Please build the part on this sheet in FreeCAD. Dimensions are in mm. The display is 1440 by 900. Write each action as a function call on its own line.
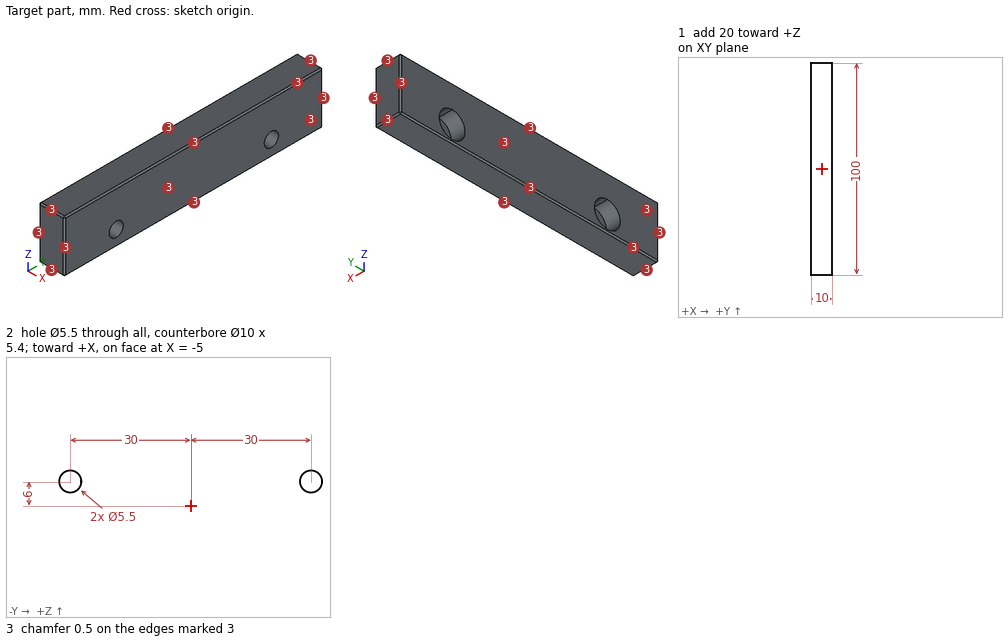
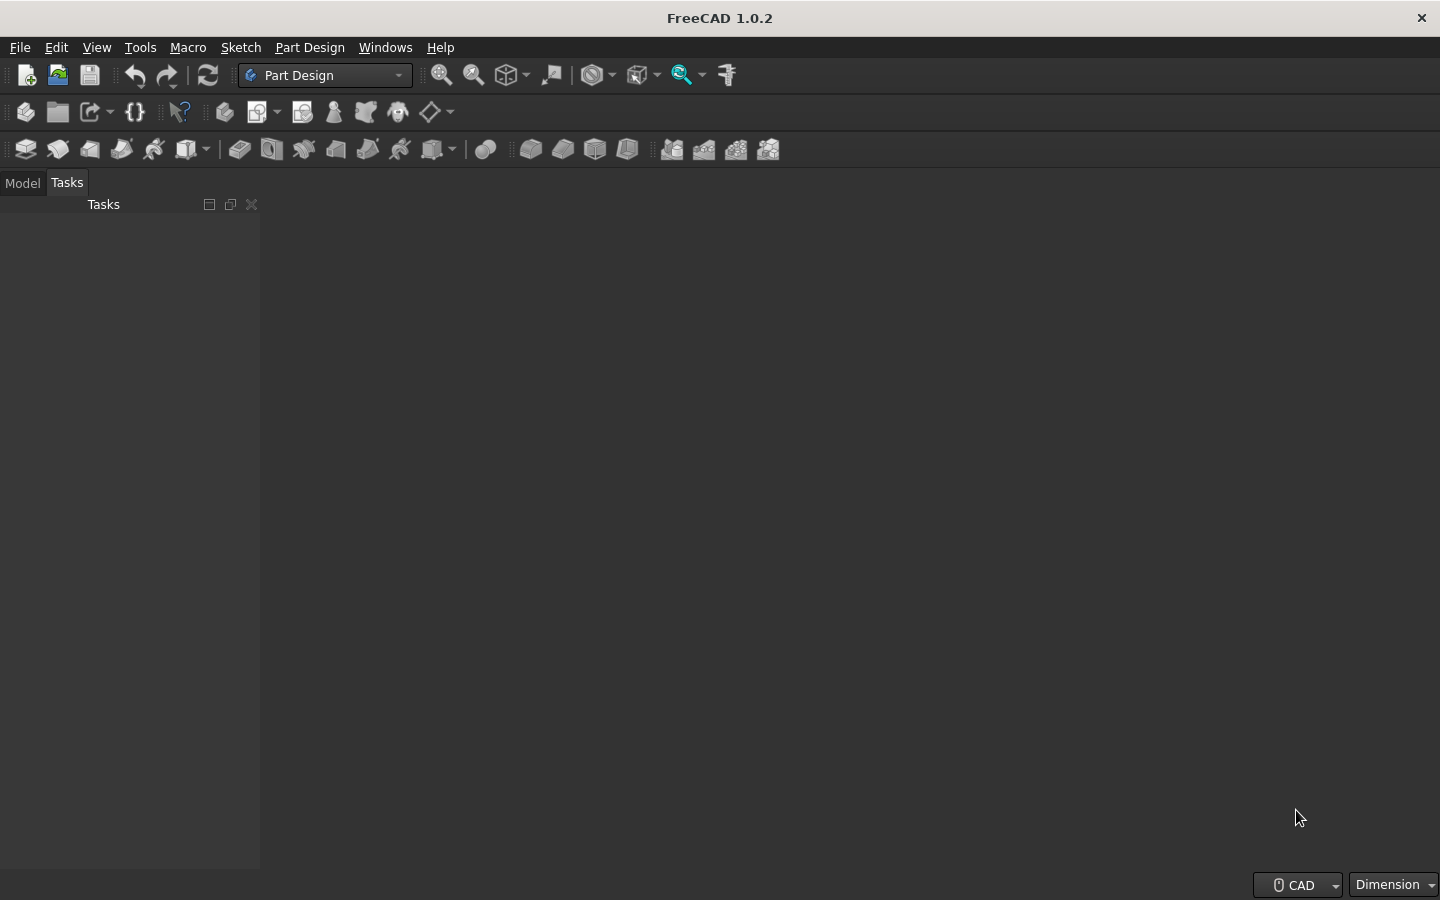
click(26, 76)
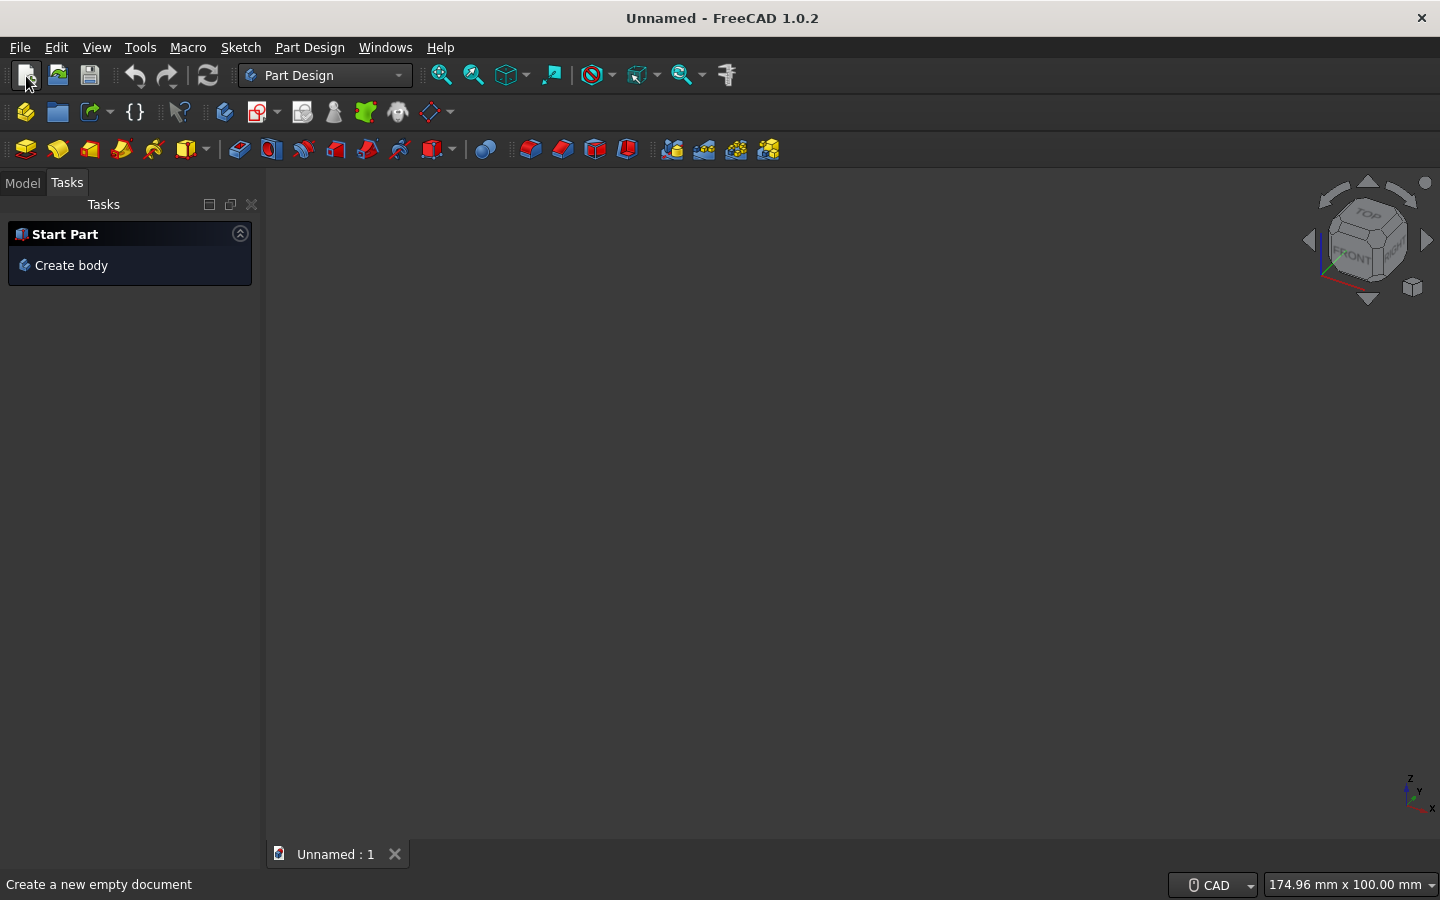
click(258, 112)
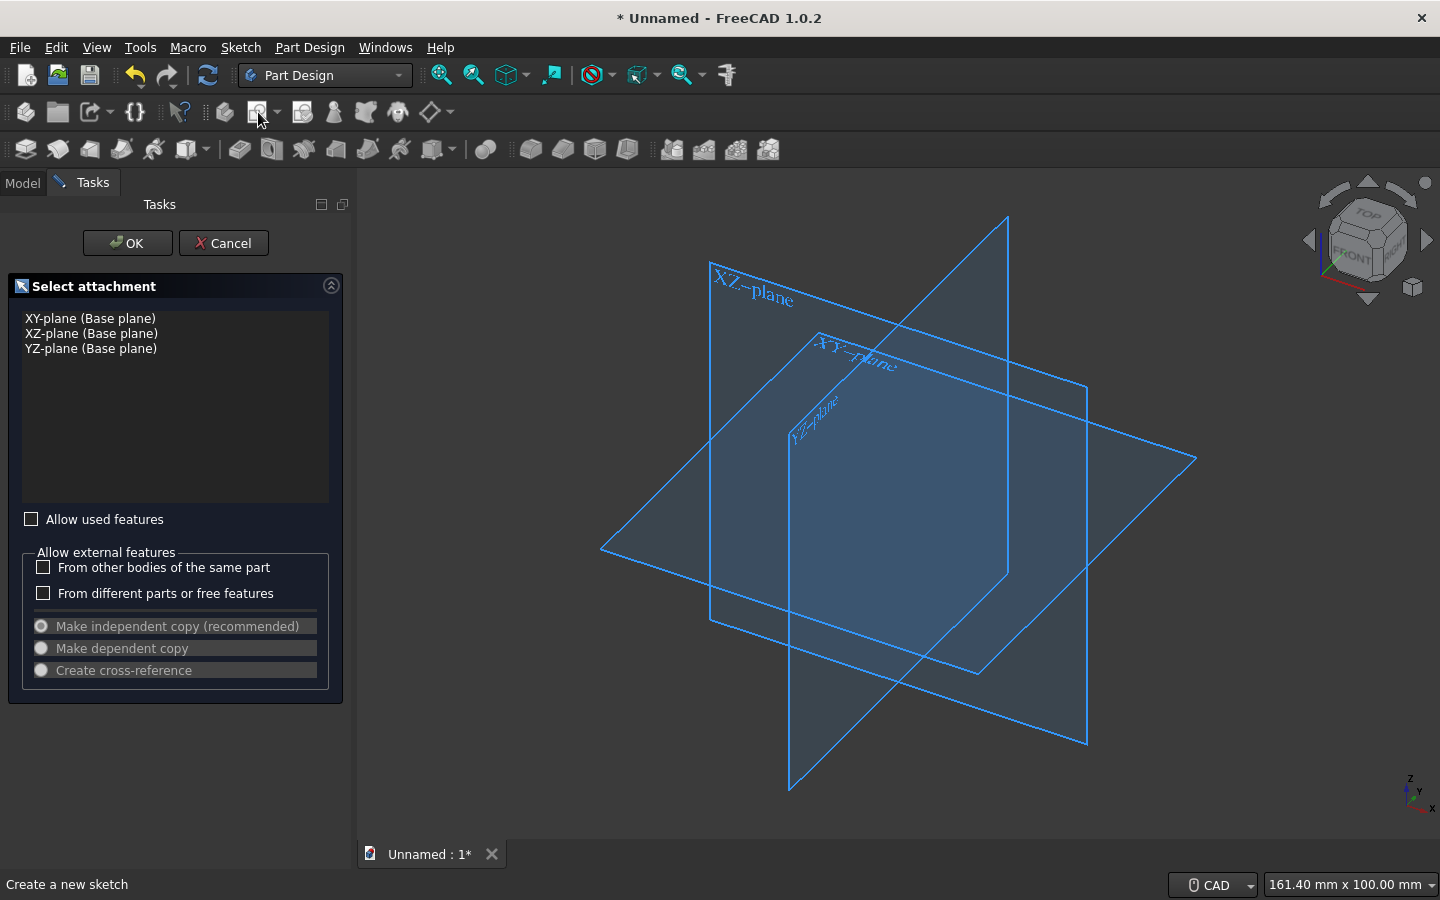
click(82, 318)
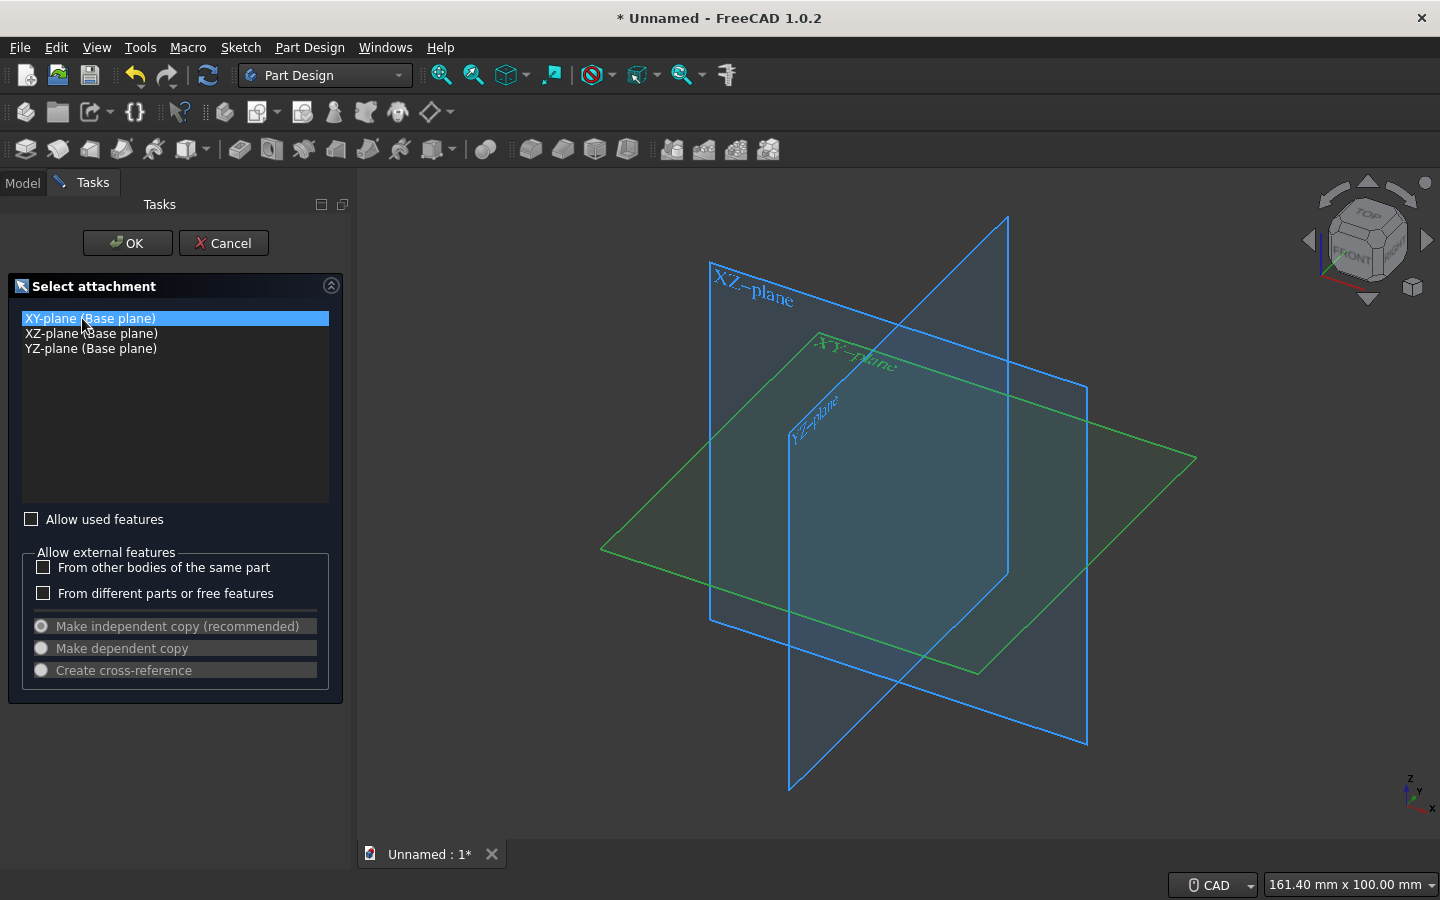
click(128, 243)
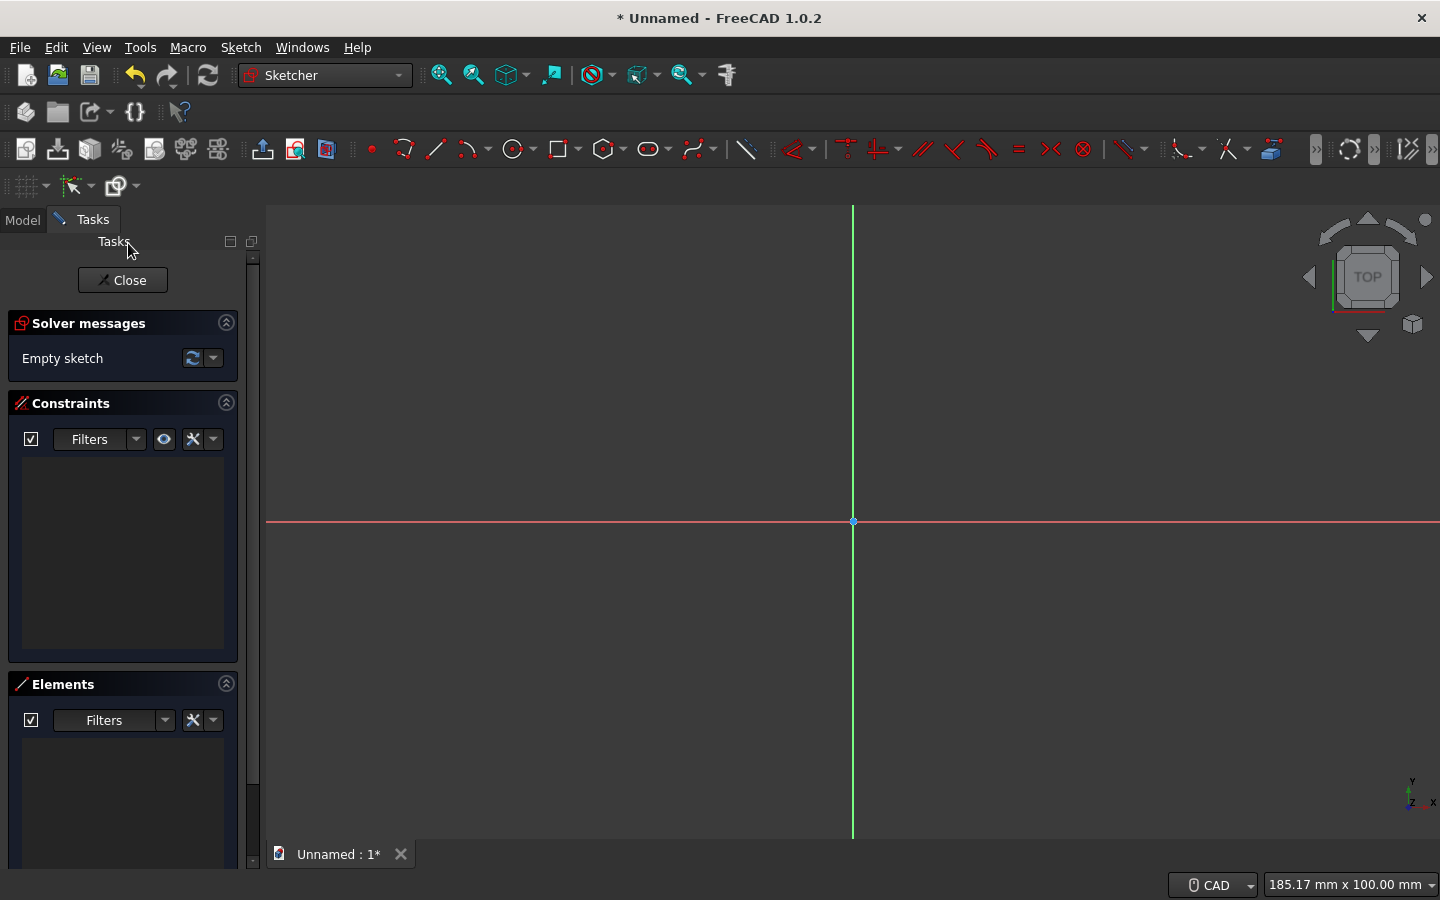
scroll(645, 522, down, 2)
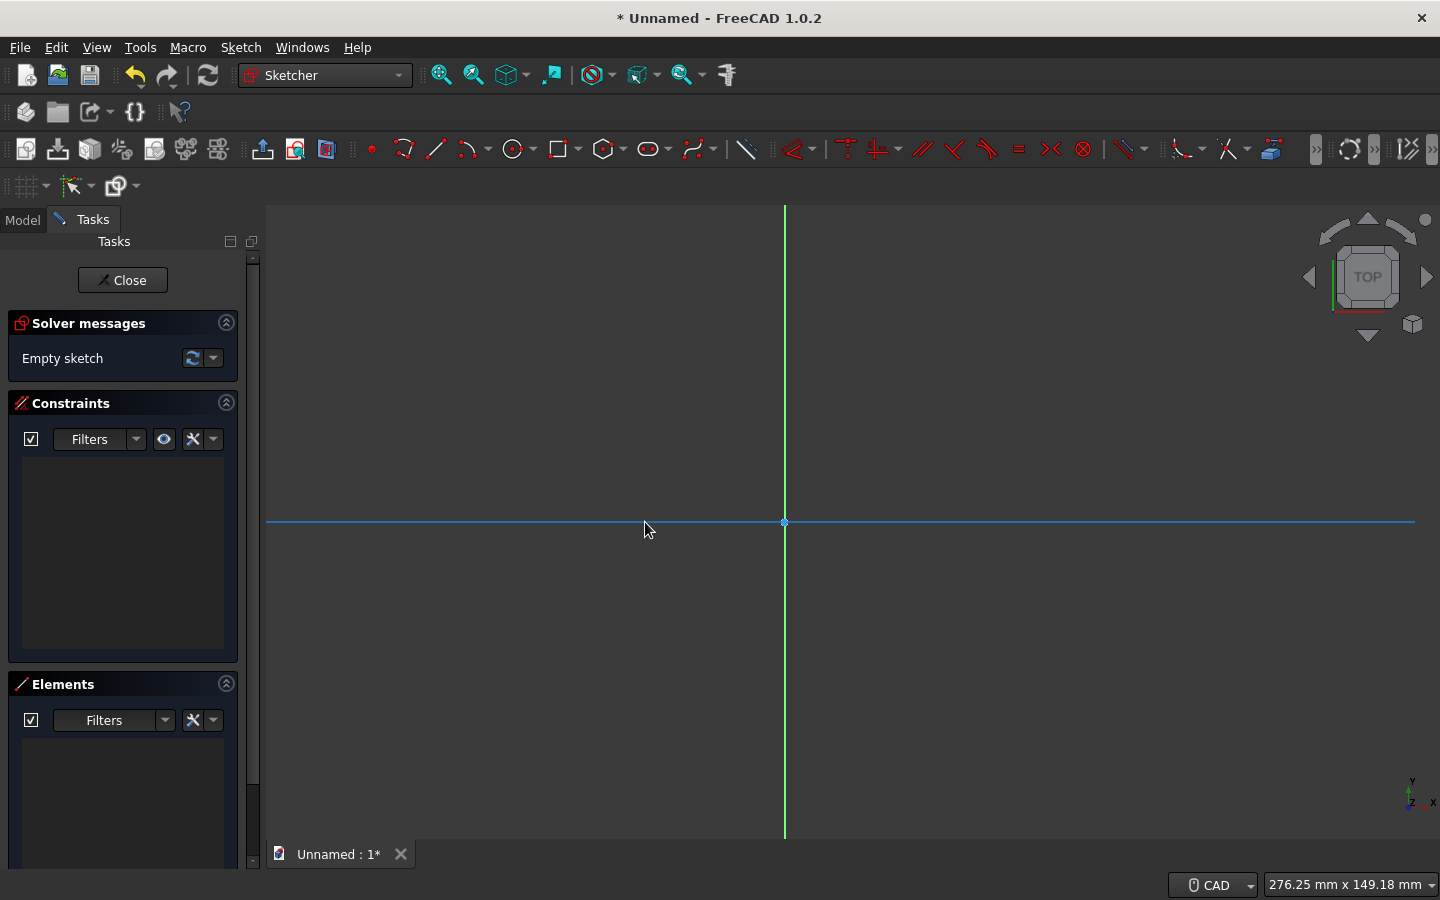
click(580, 150)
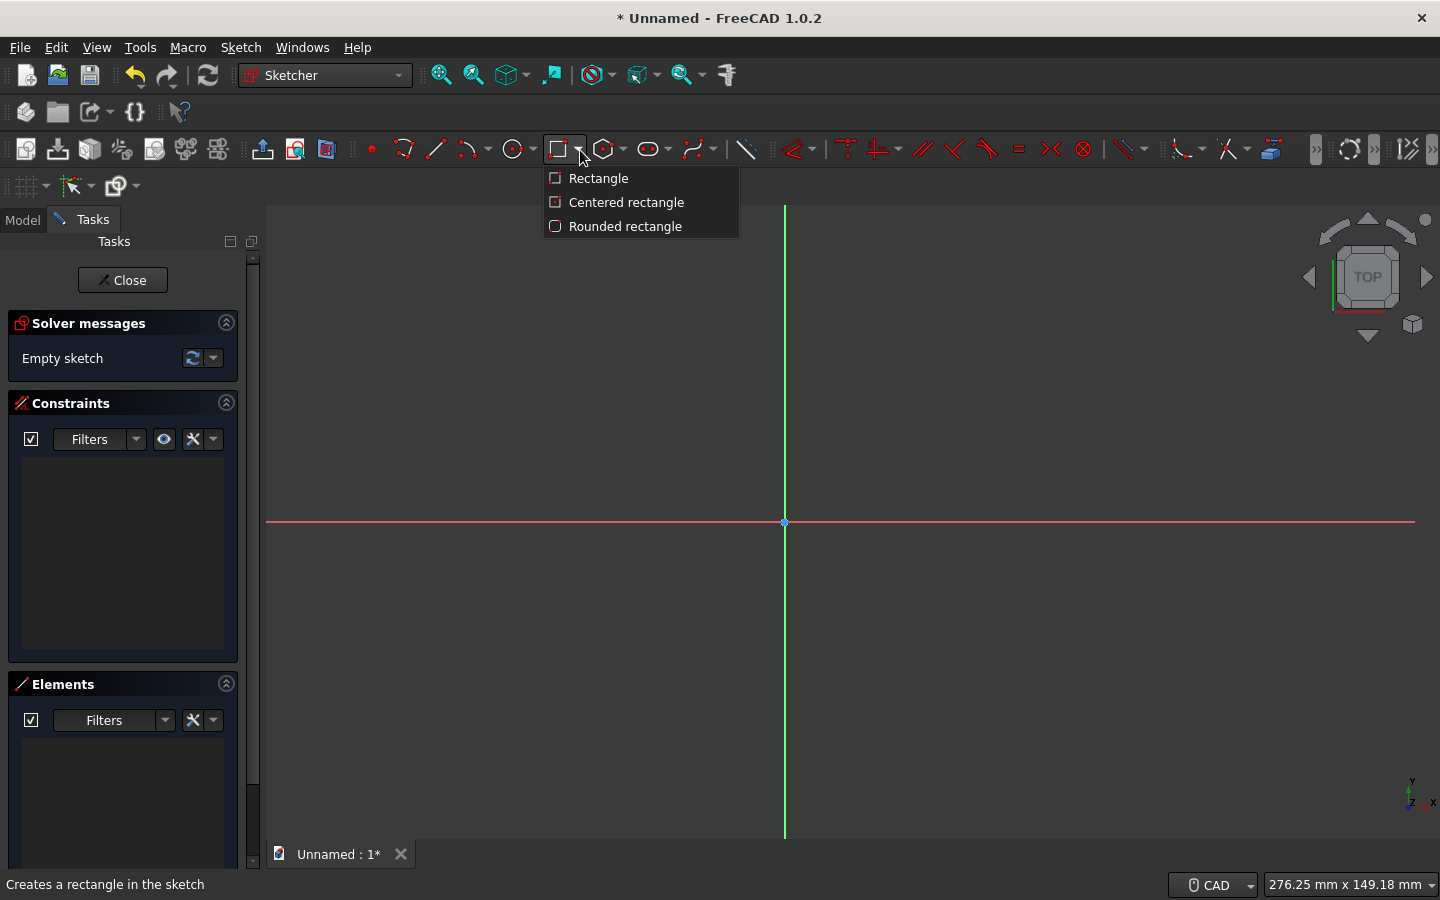
click(642, 202)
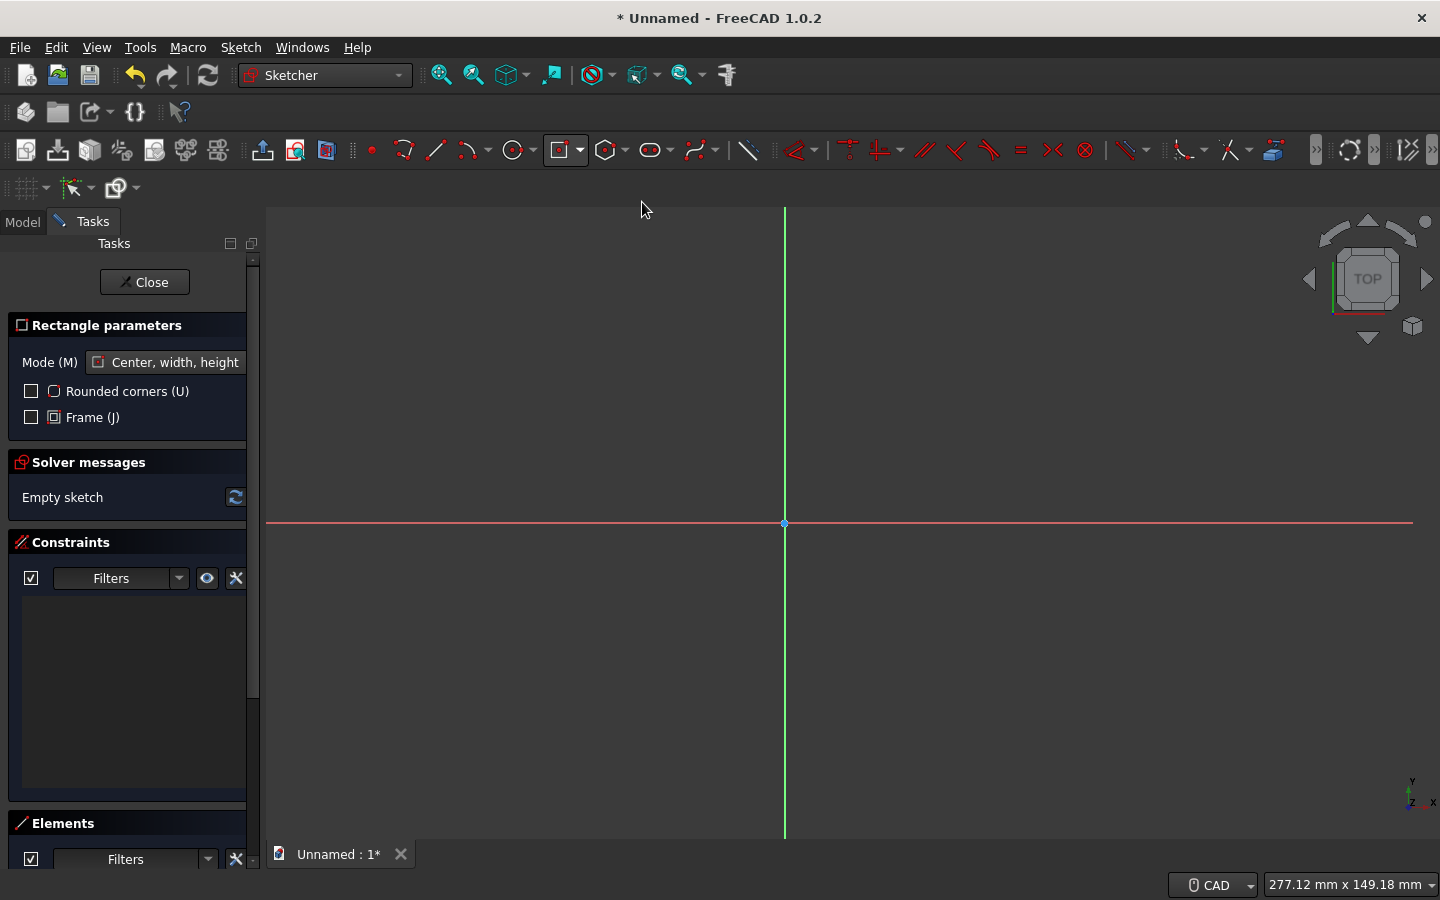
click(785, 523)
click(806, 311)
key(Escape)